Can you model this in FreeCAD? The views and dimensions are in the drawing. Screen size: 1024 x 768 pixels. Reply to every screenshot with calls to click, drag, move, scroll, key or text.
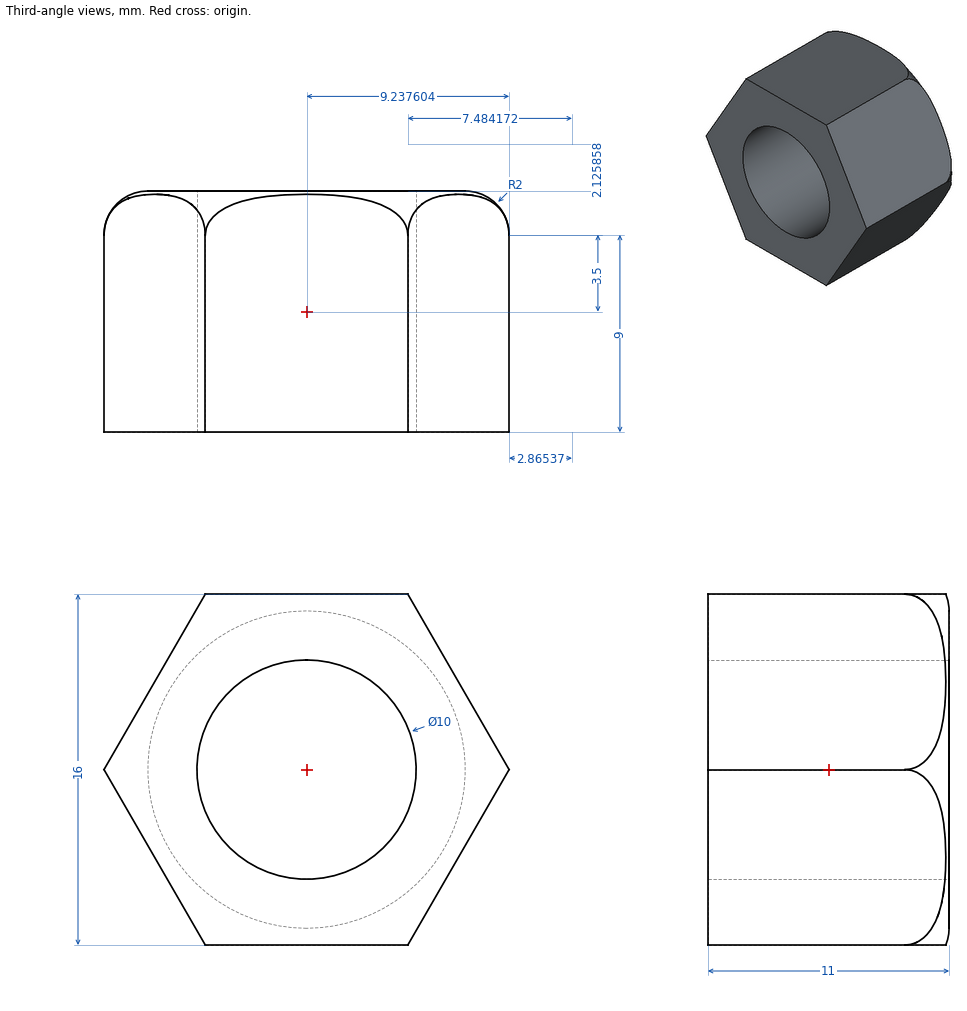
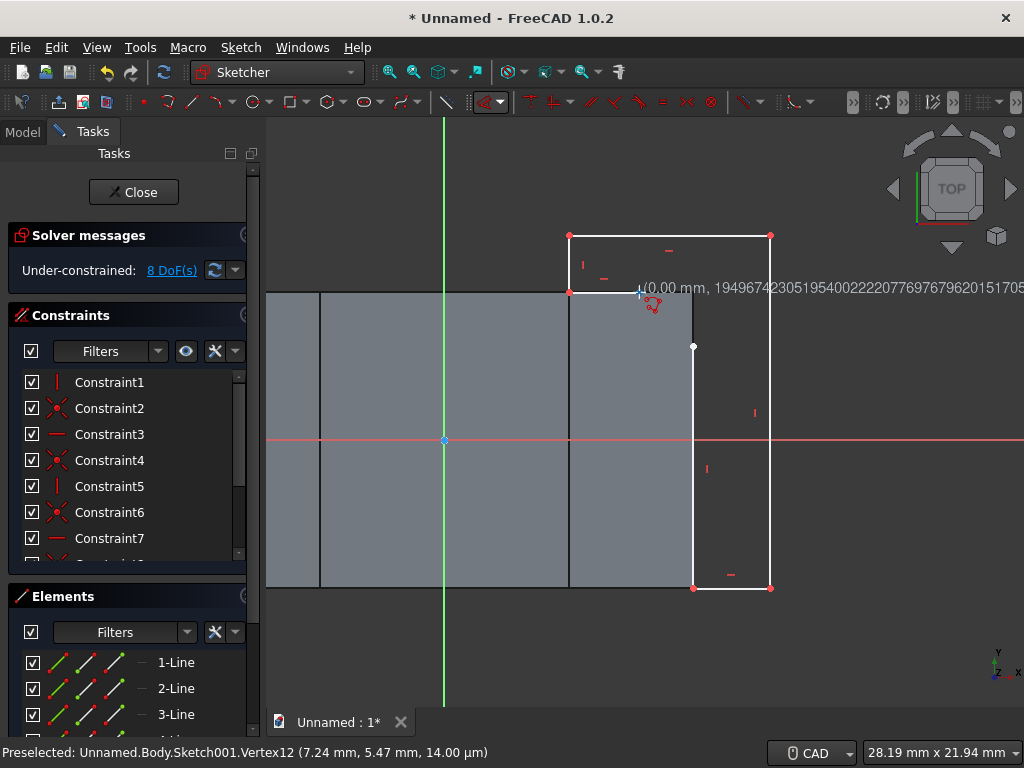
key(g)
key(3)
key(a)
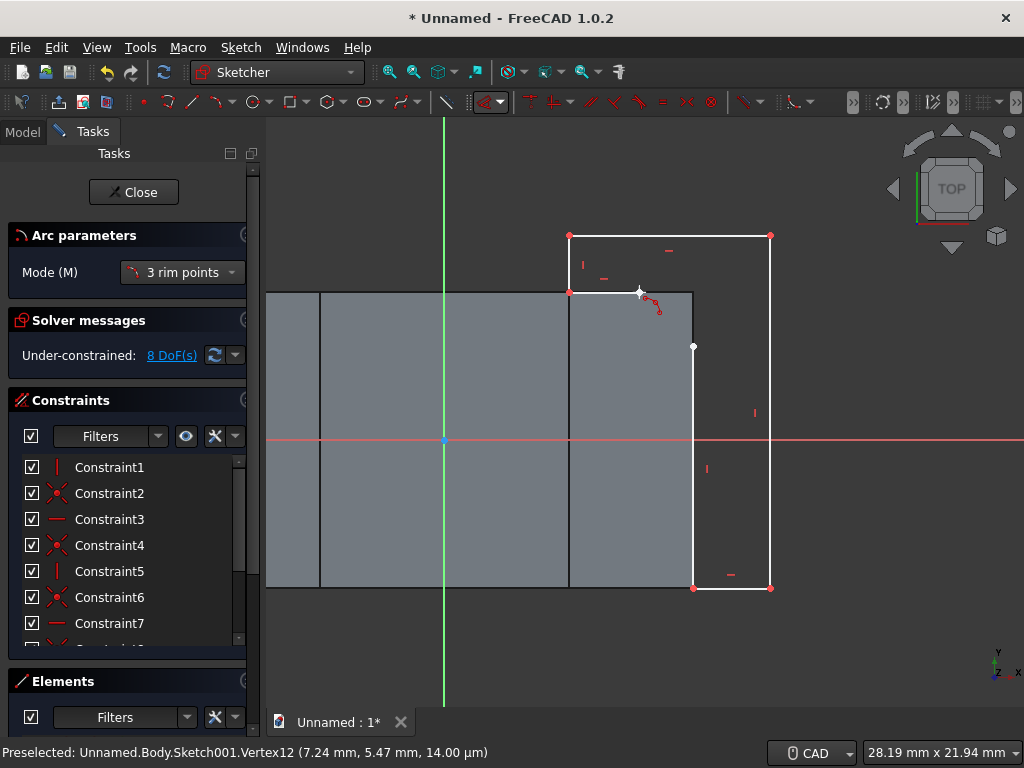
click(639, 293)
click(693, 347)
click(677, 308)
key(Escape)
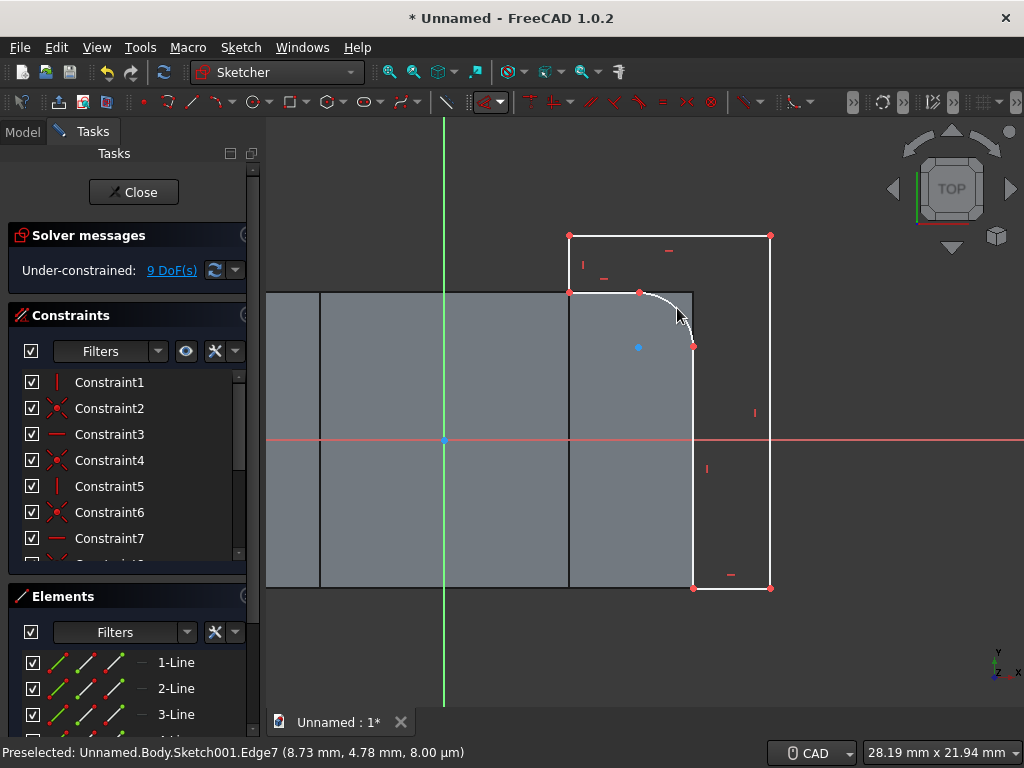
click(693, 420)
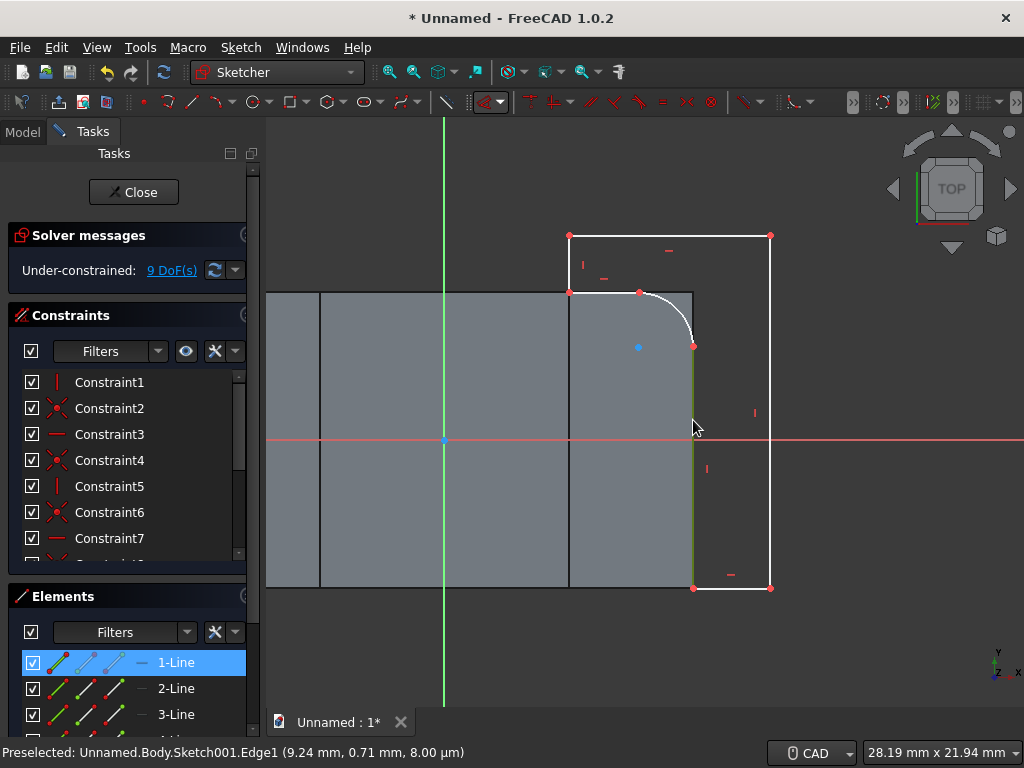
click(687, 323)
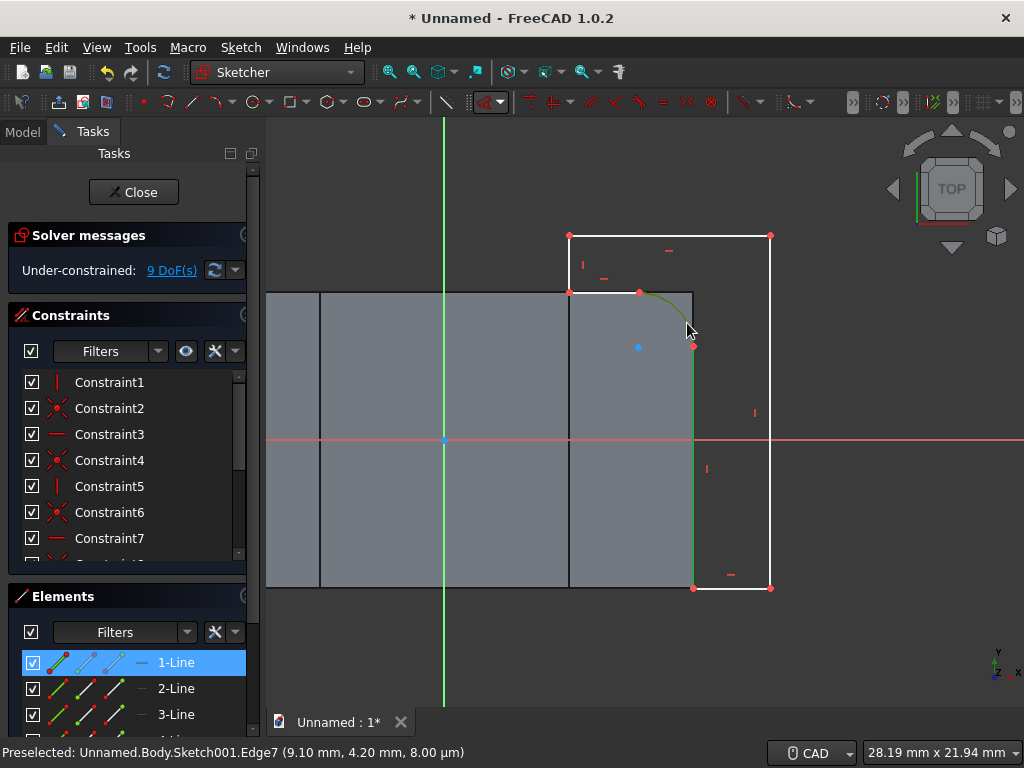
click(640, 102)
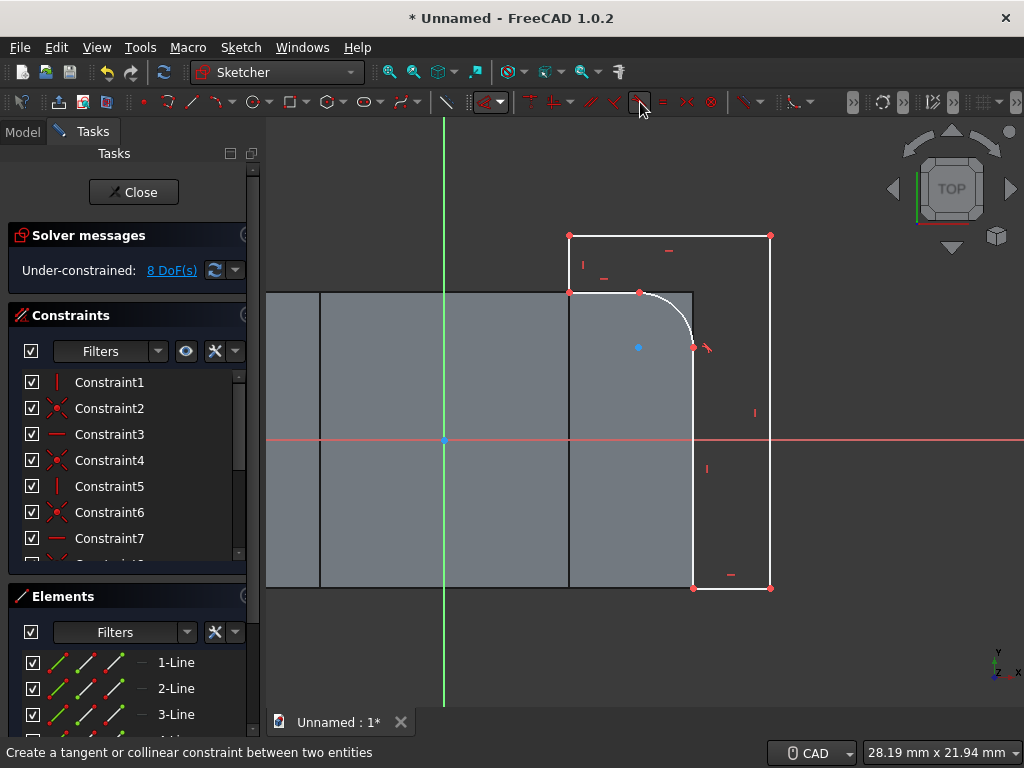
click(590, 293)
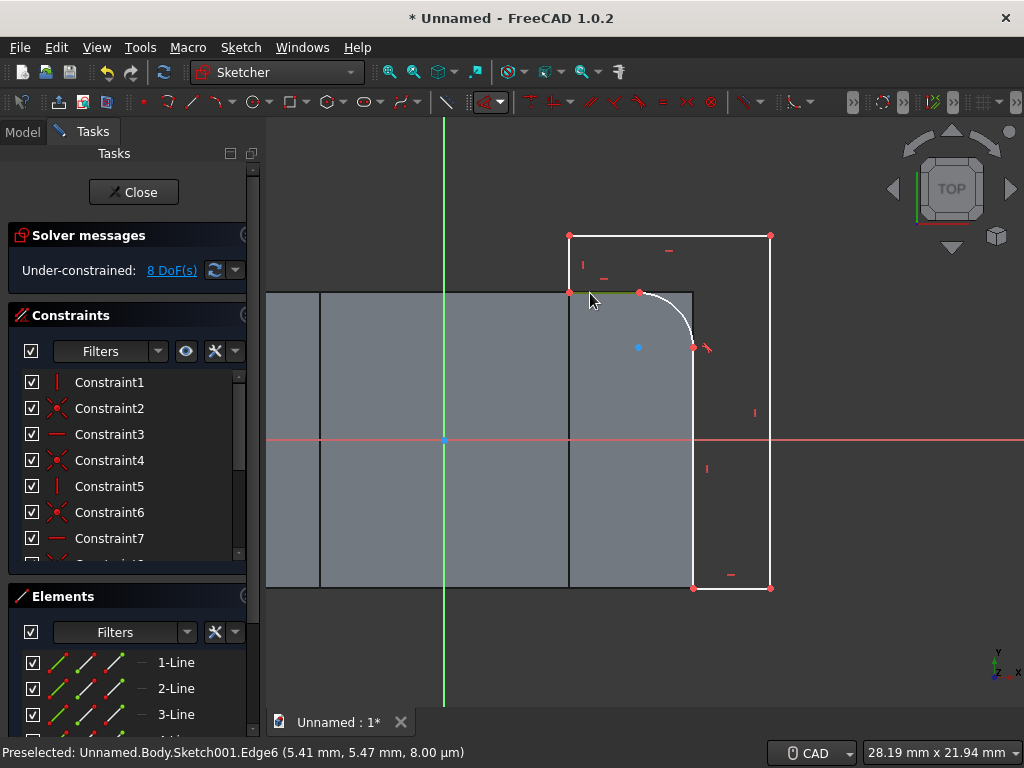
click(687, 323)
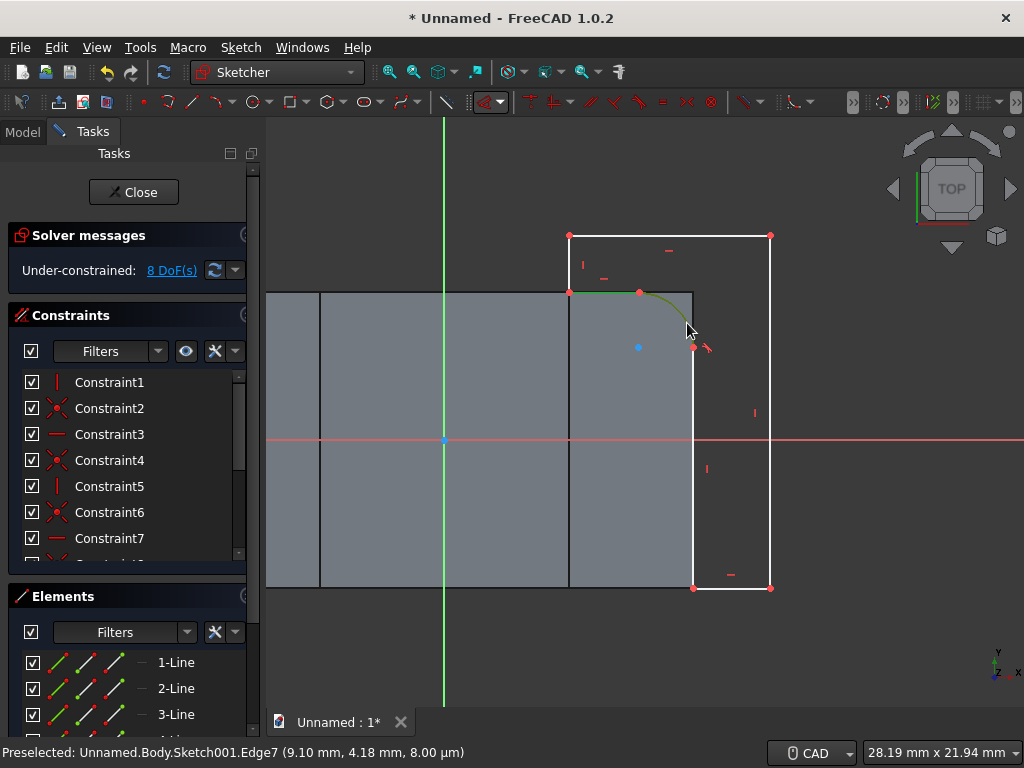
key(t)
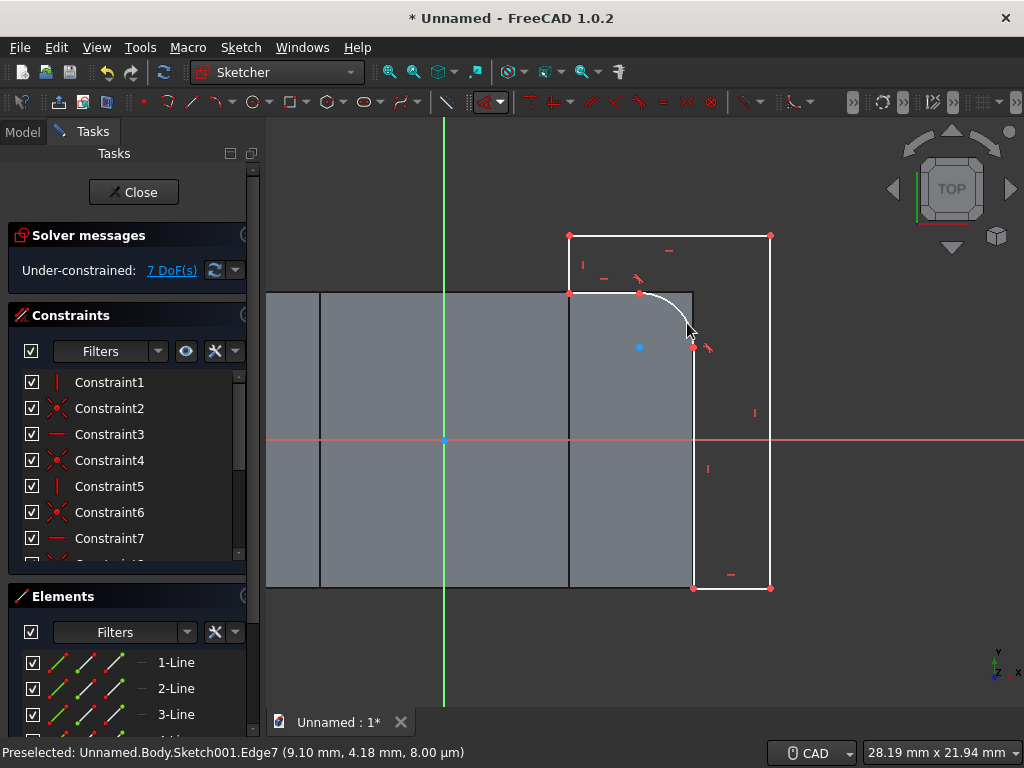
click(688, 323)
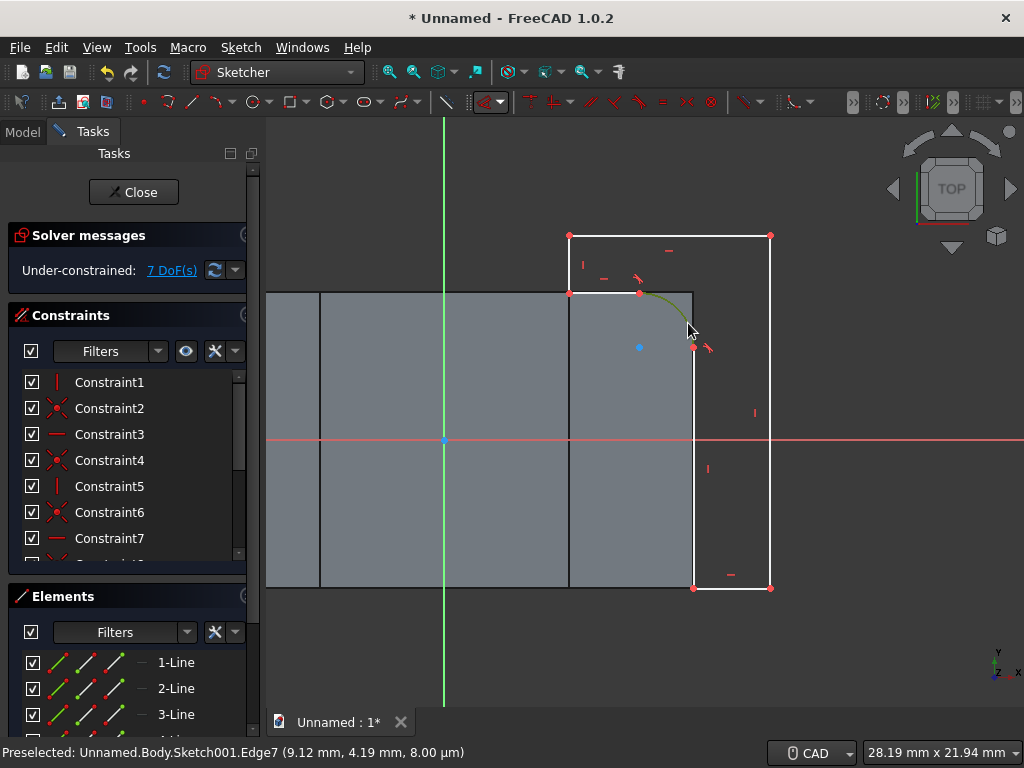
click(502, 102)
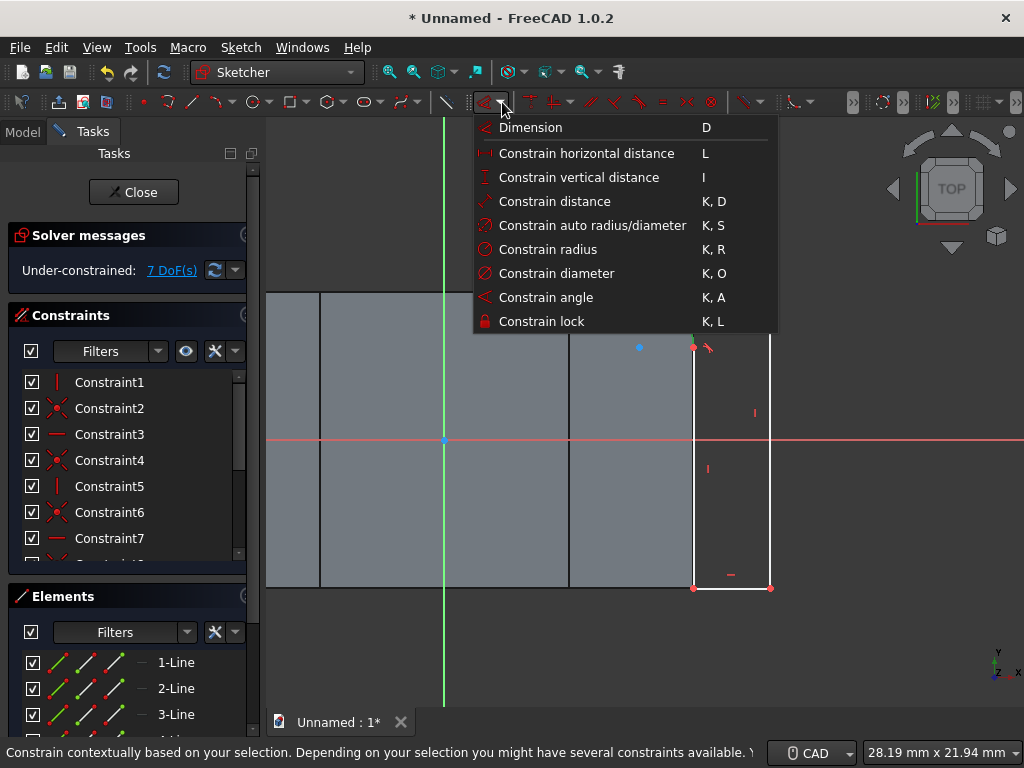
click(626, 249)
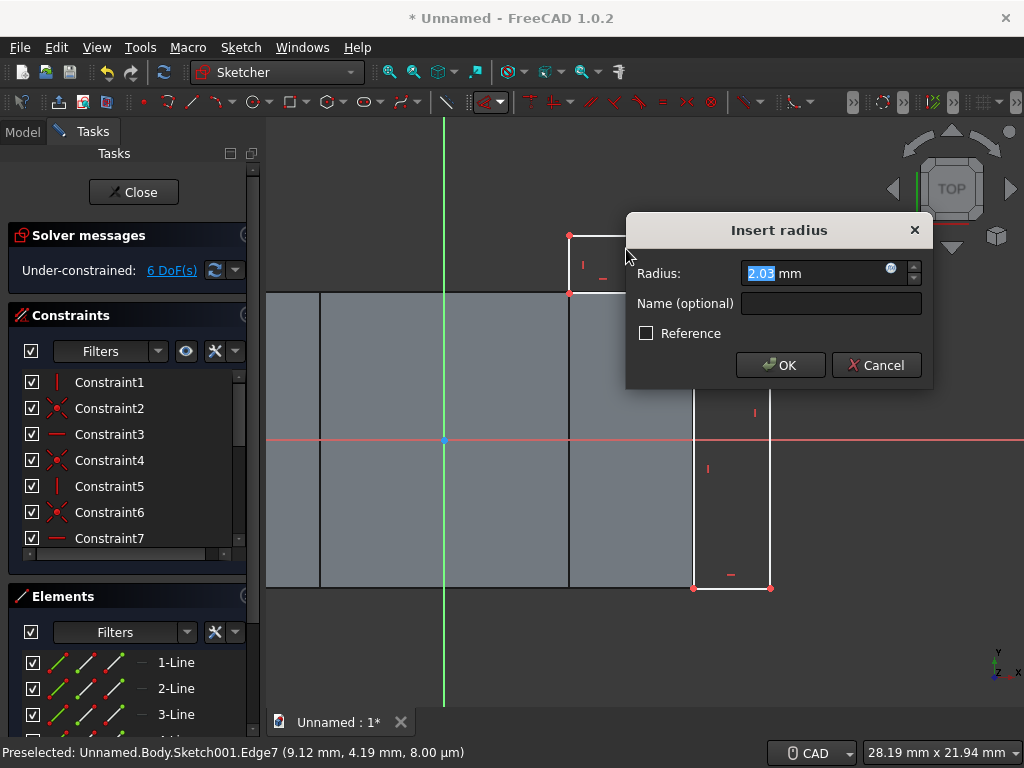
text(2)
key(Return)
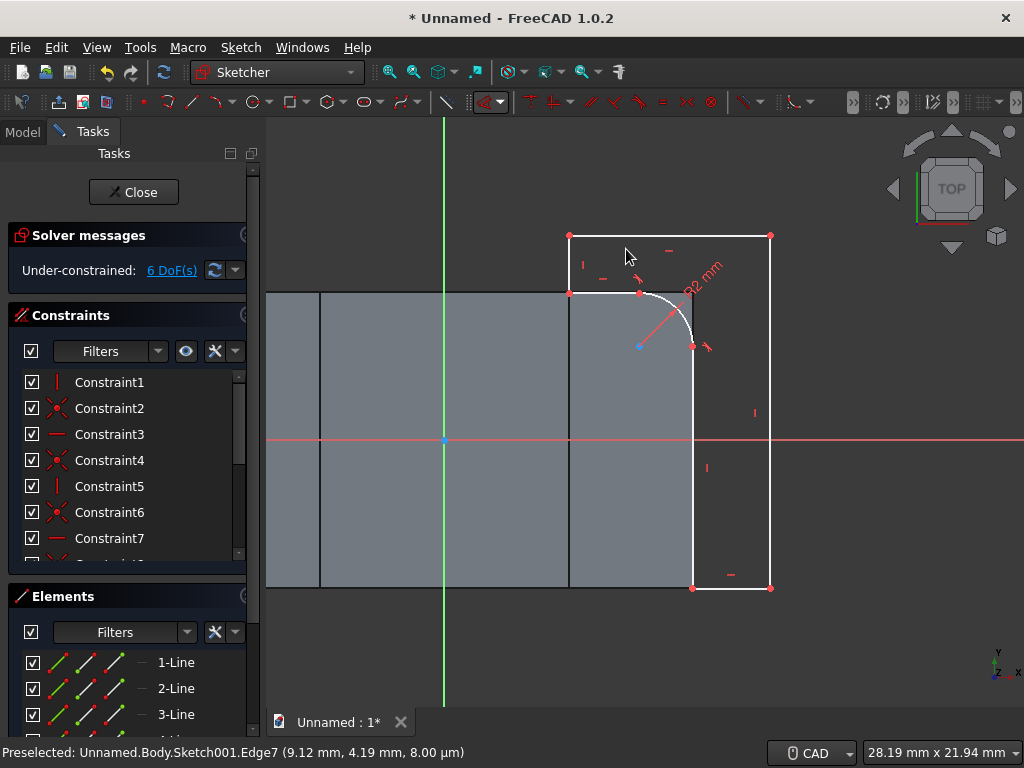
click(693, 419)